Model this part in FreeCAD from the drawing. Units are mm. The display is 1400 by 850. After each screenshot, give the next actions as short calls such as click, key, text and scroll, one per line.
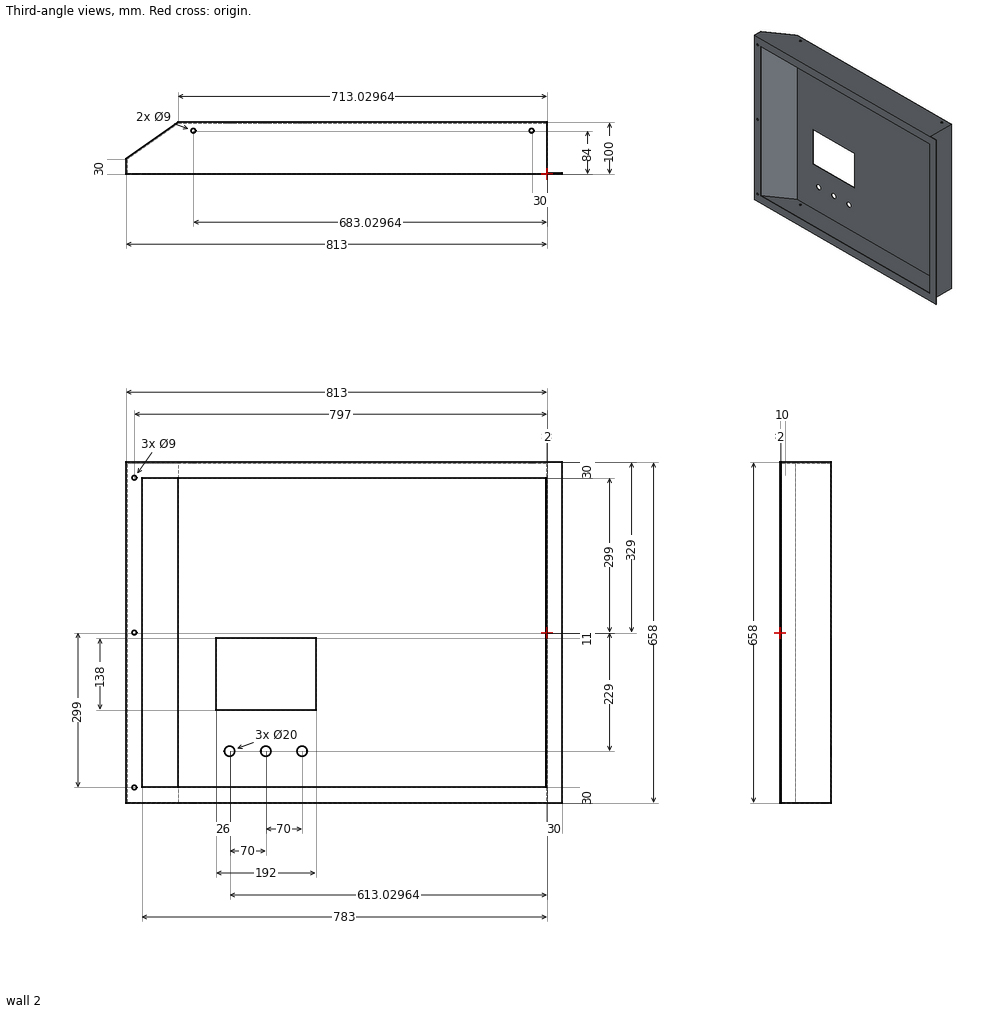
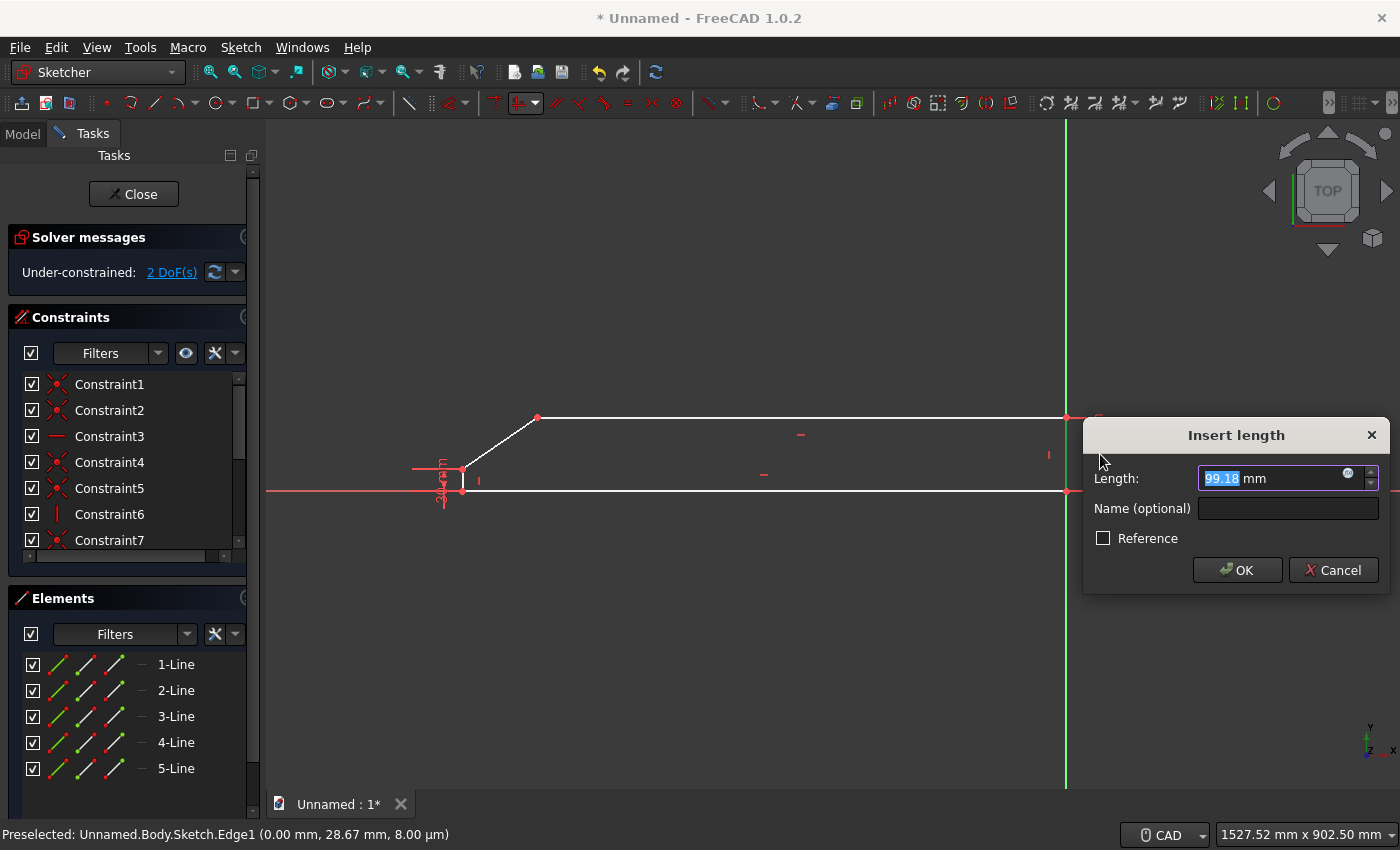
text(100)
key(Return)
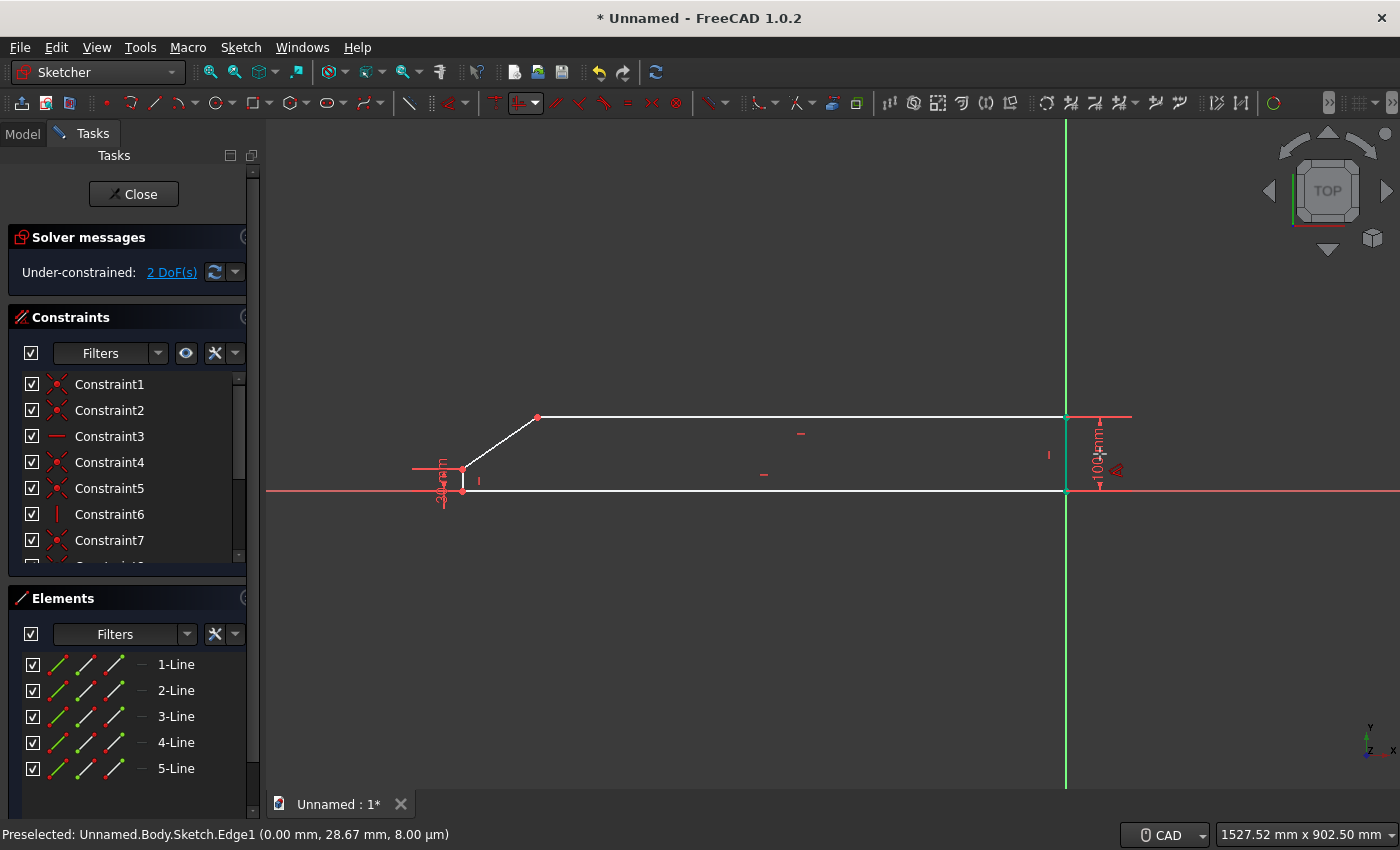
click(644, 491)
click(765, 525)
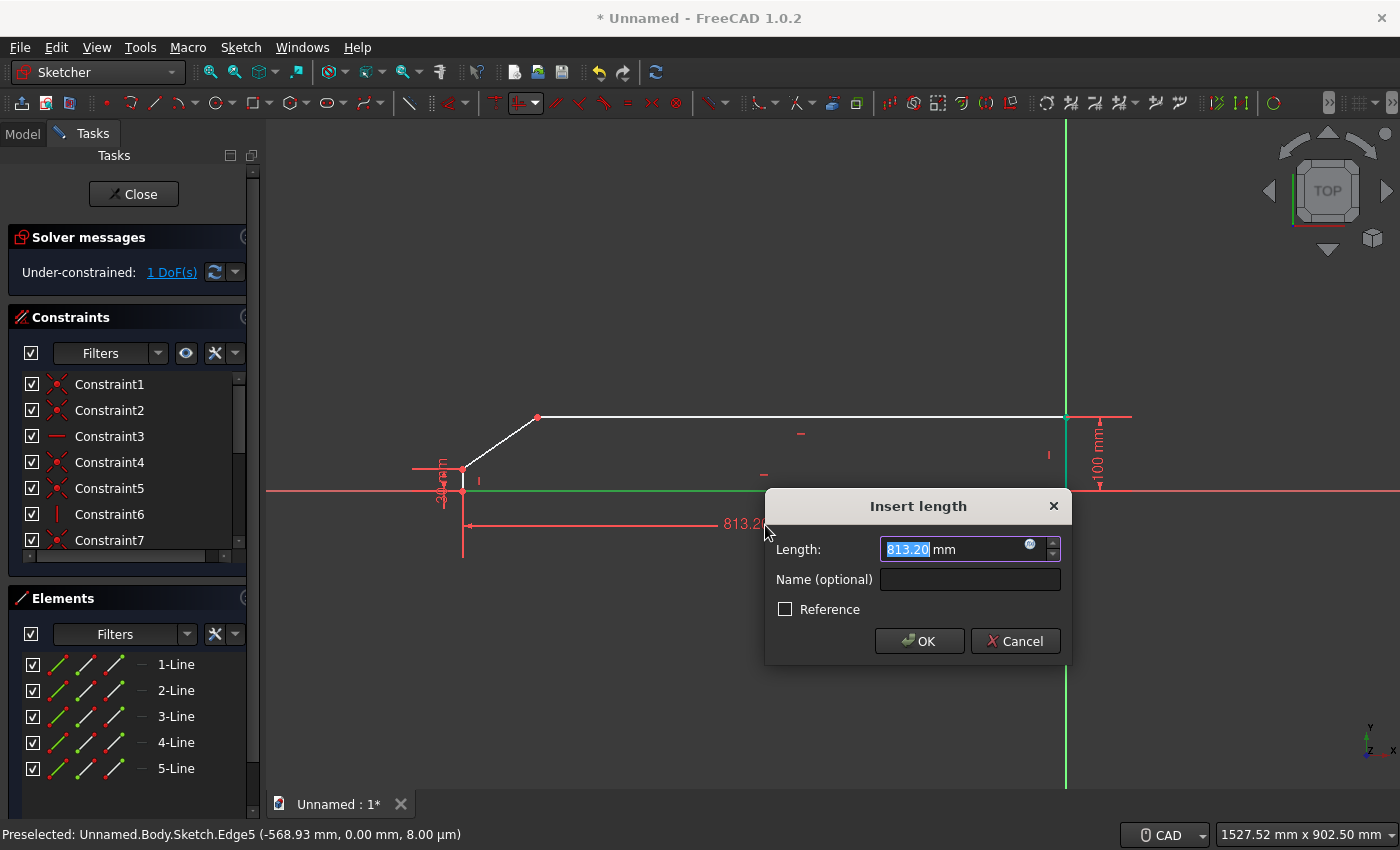
text(813)
key(Return)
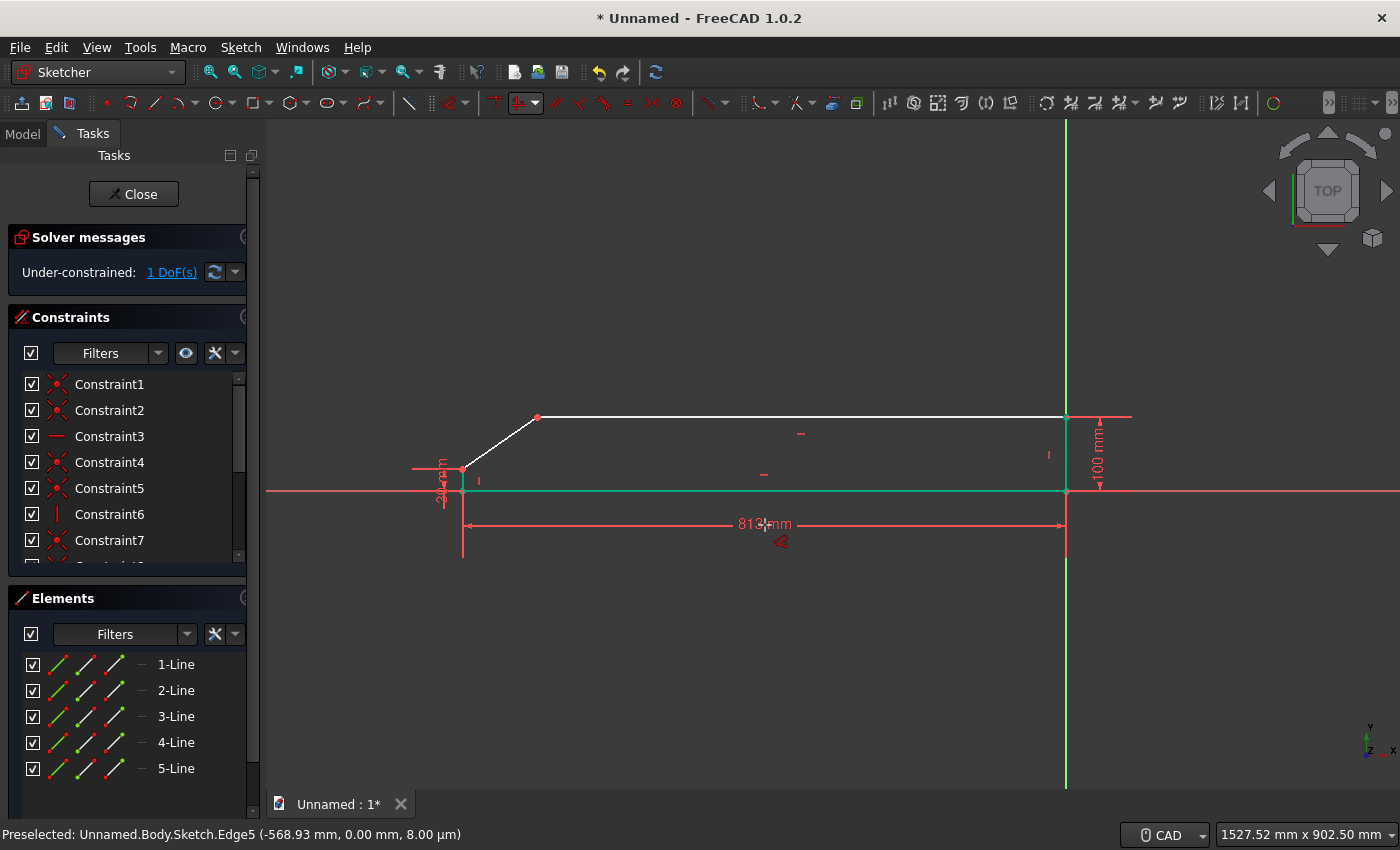
click(908, 417)
click(802, 383)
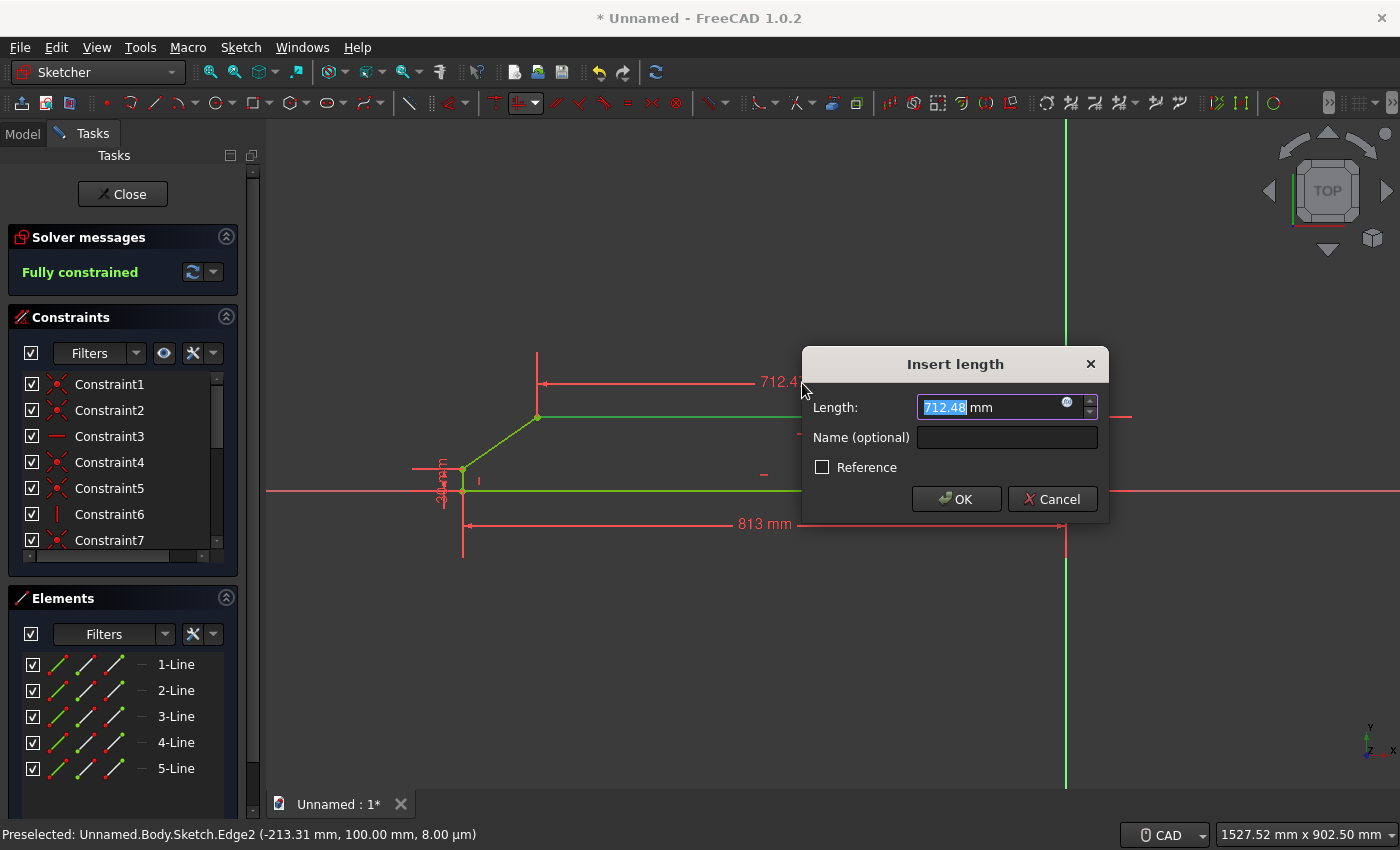
text(713.02964)
key(Return)
key(Escape)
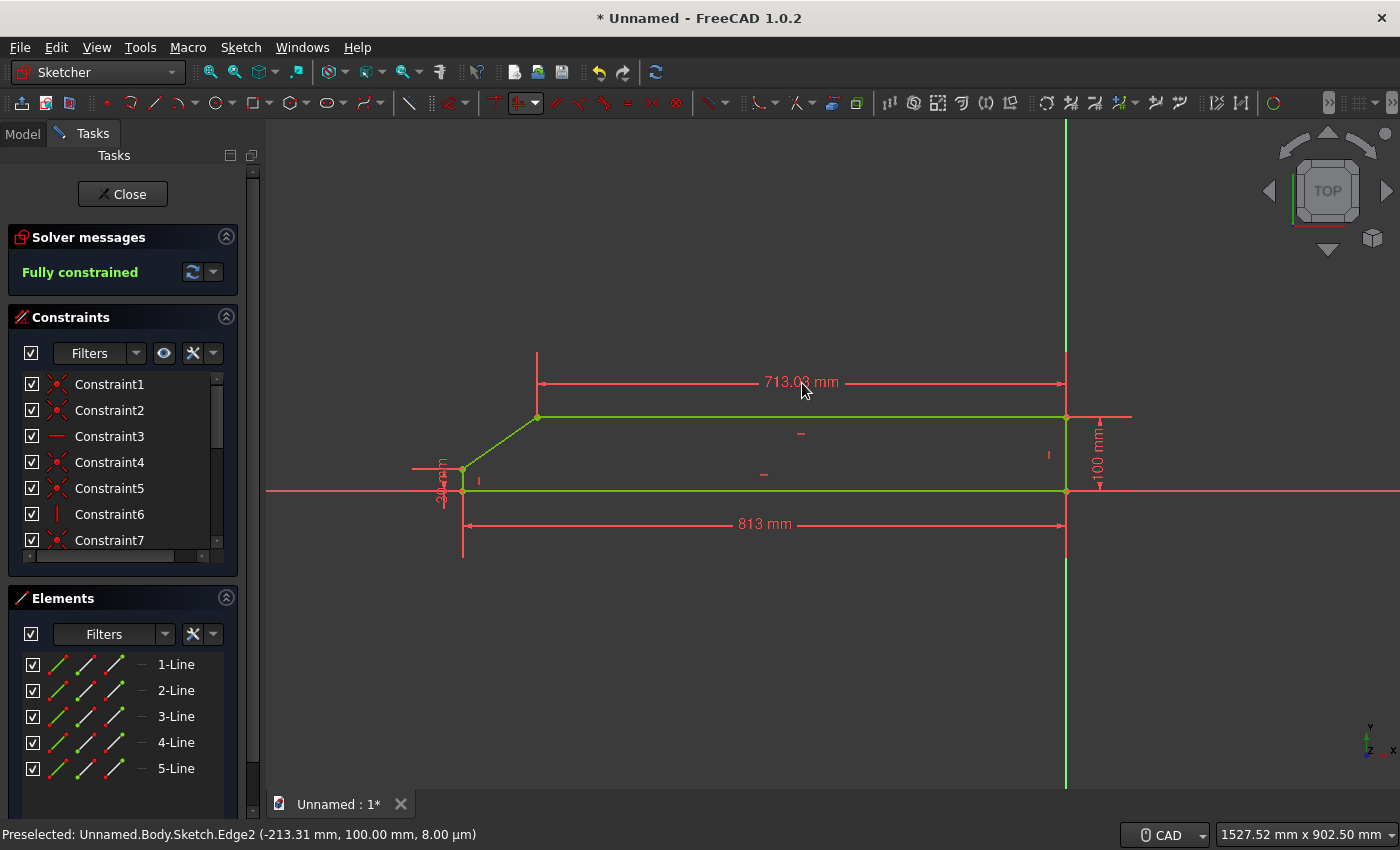
click(123, 194)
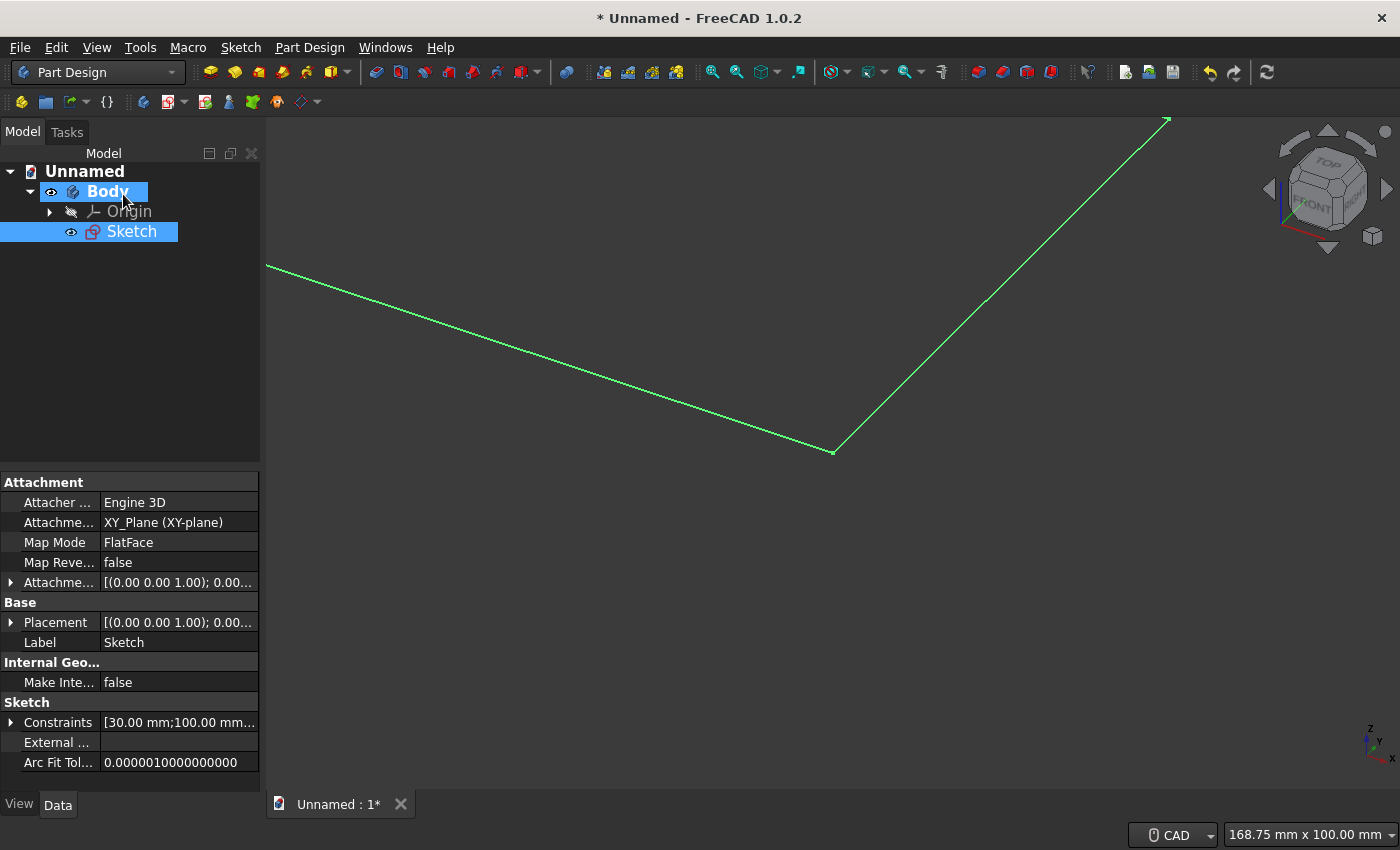
click(212, 72)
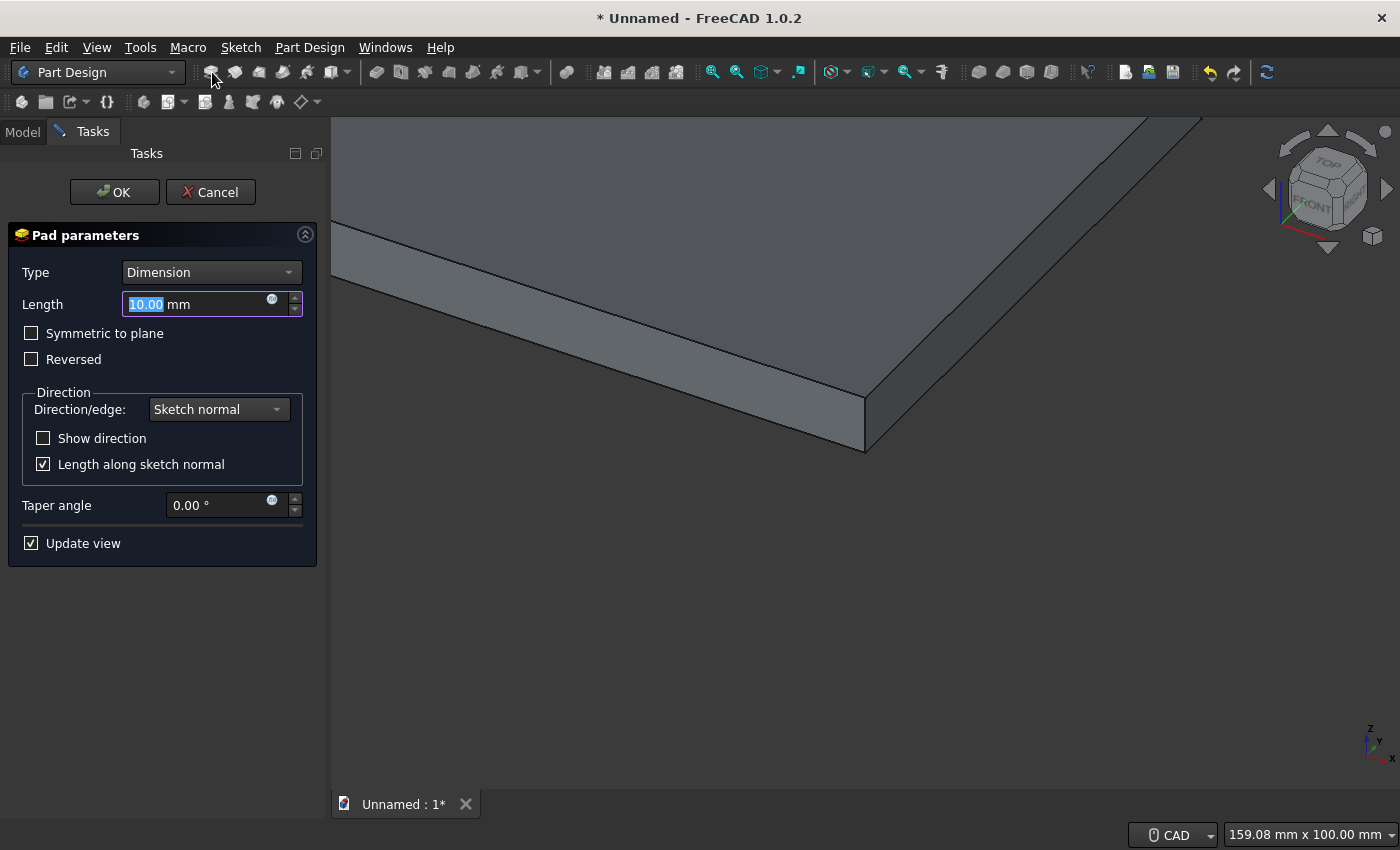
text(658)
key(Tab)